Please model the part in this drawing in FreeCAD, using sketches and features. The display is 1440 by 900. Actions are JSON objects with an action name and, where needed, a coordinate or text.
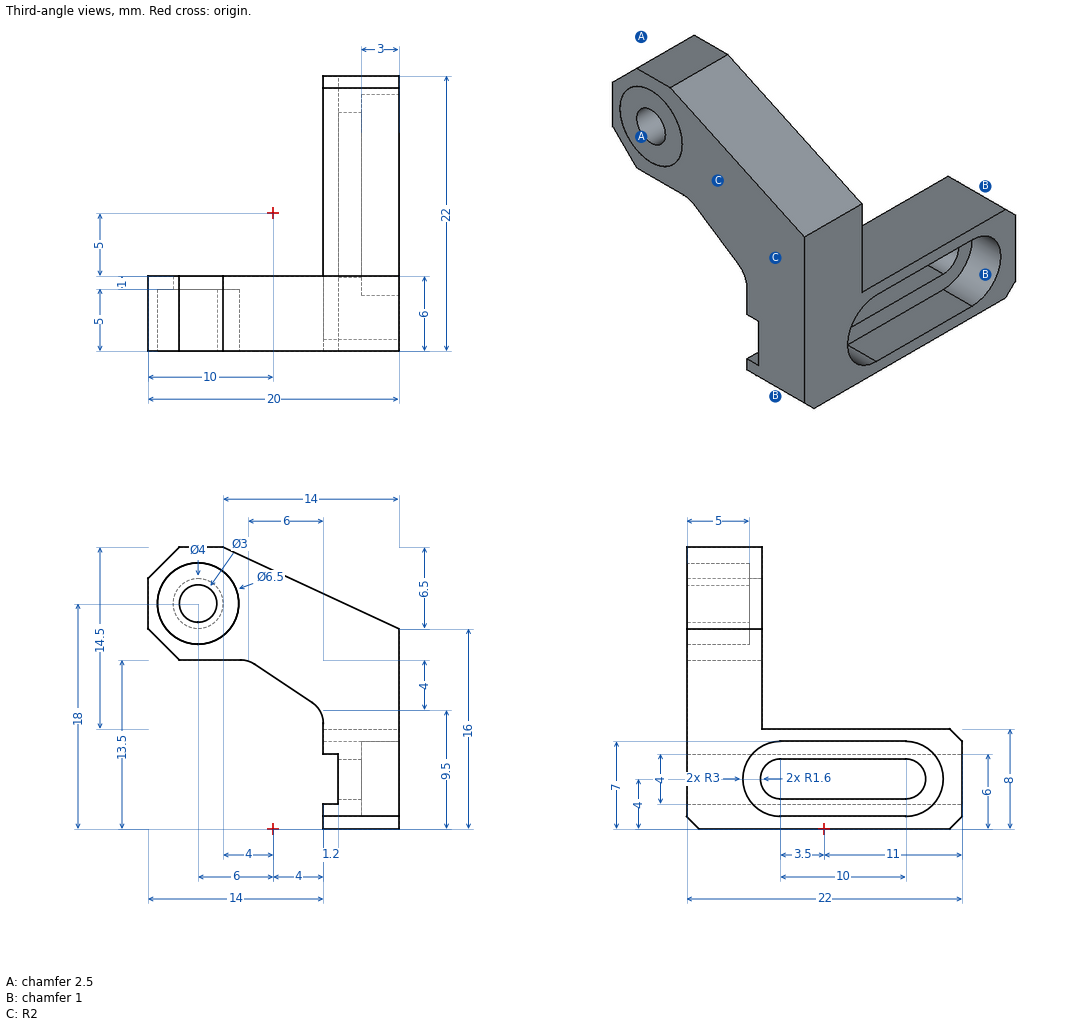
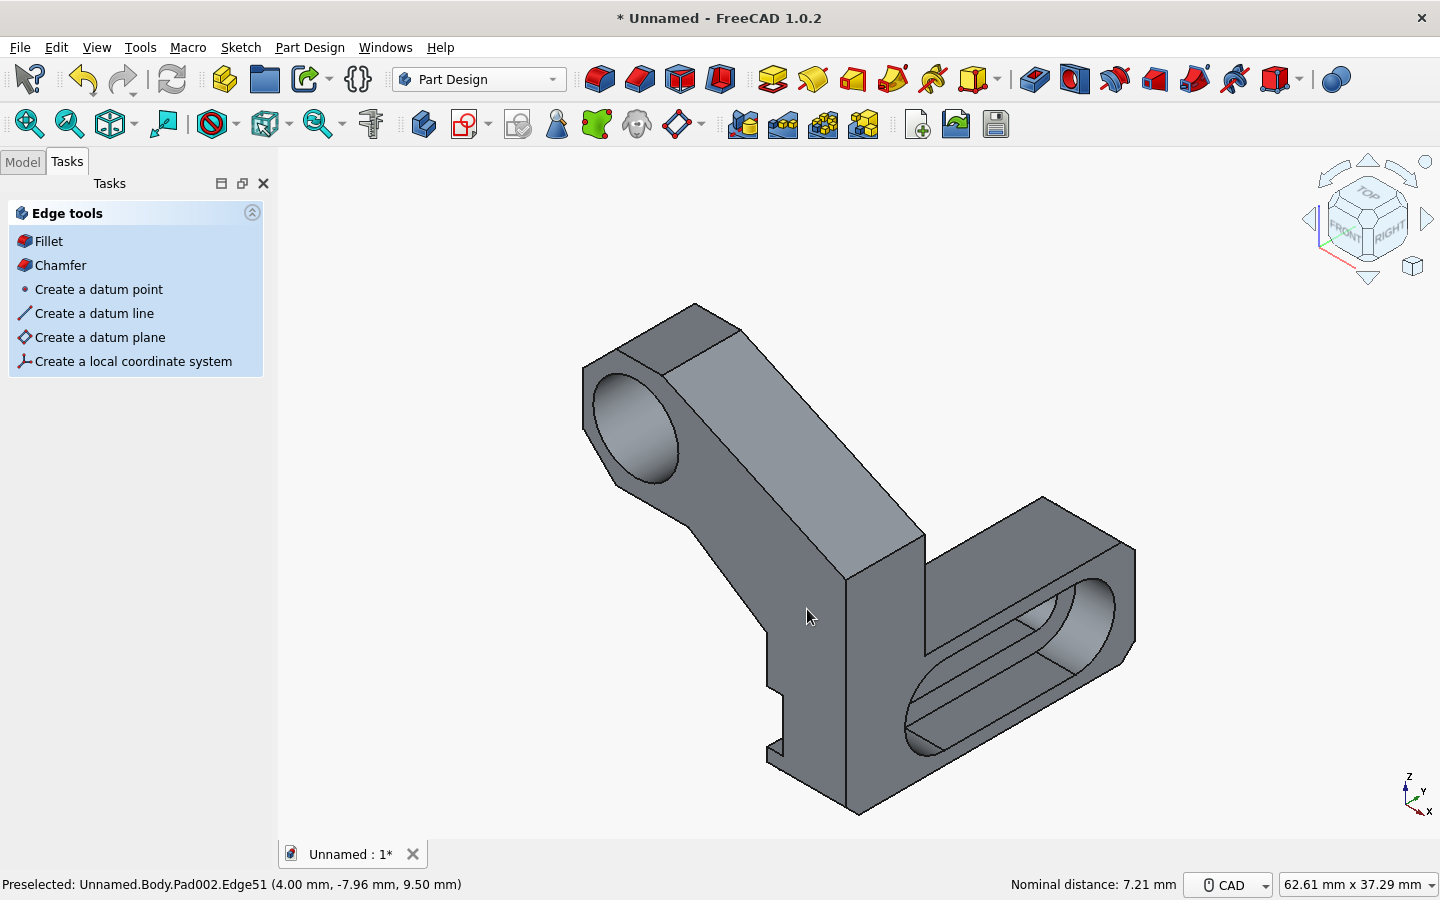
{"action": "left_click", "coordinate": [600, 80]}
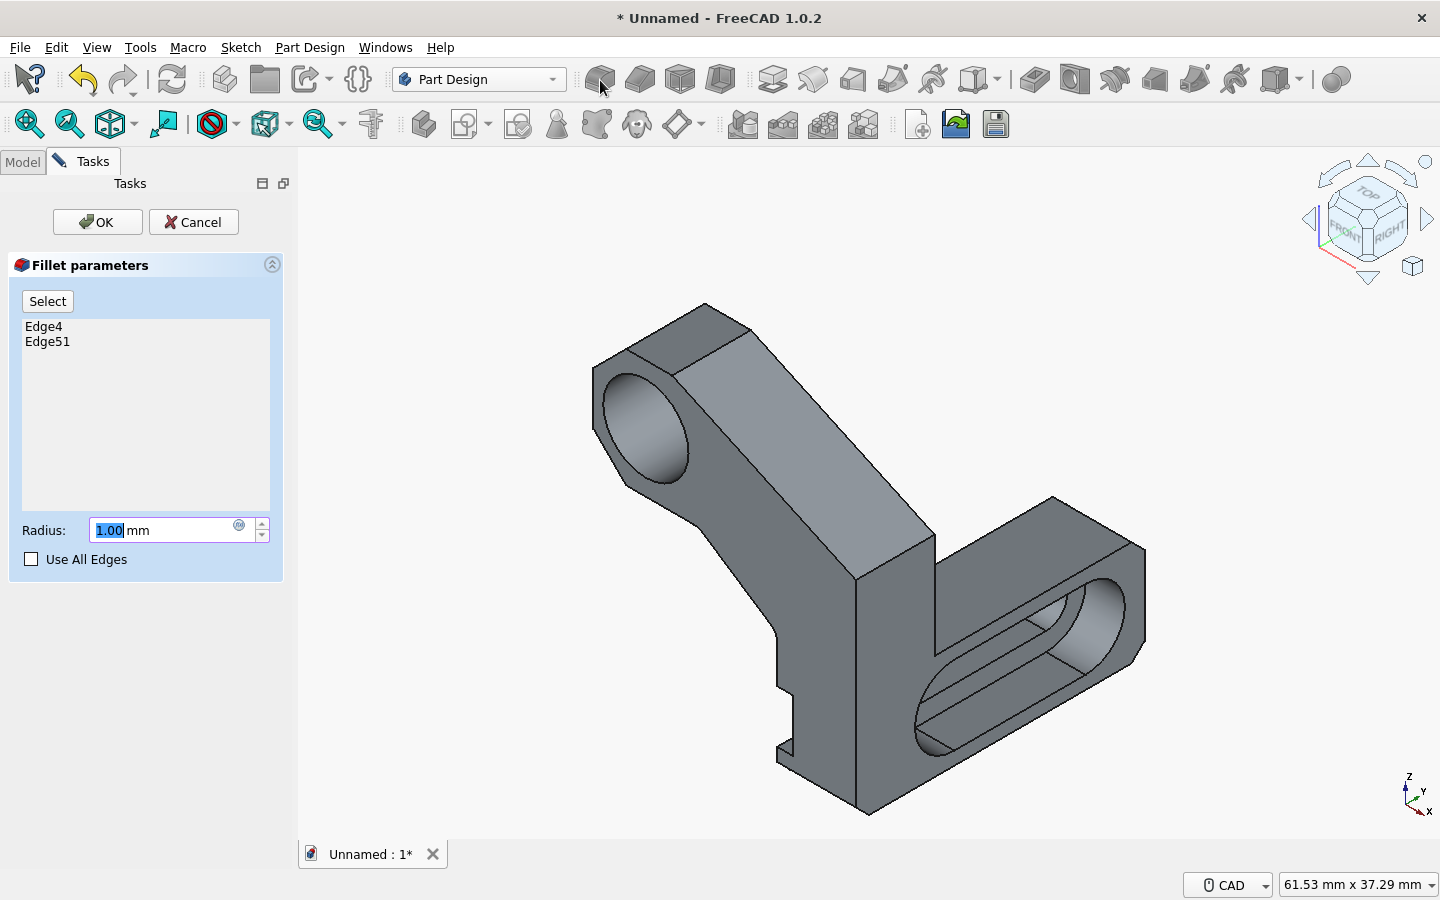
{"action": "type", "text": "2"}
{"action": "key", "text": "Tab"}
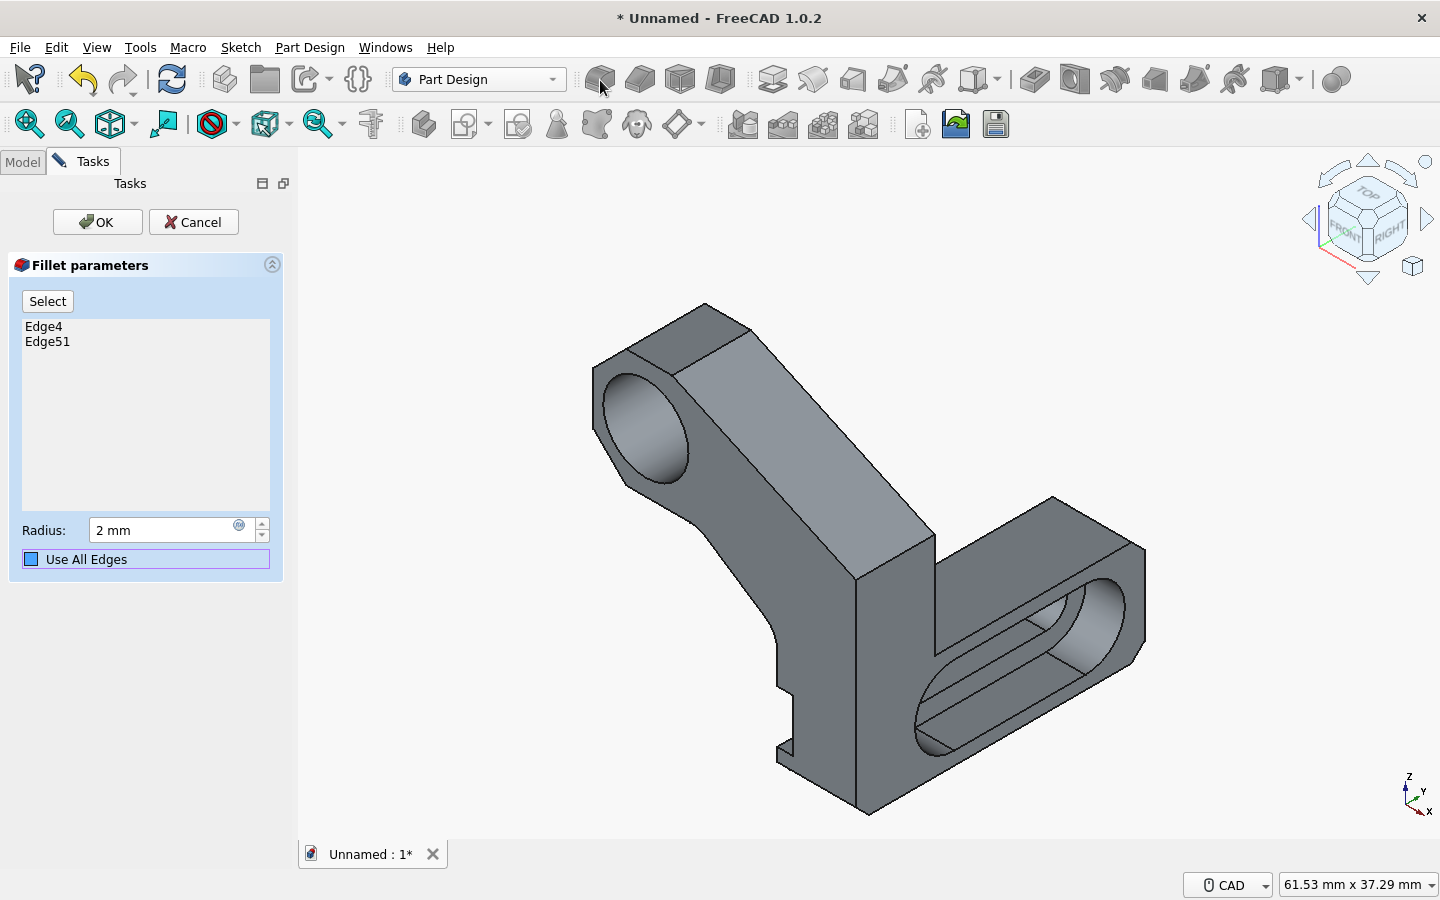
{"action": "left_click", "coordinate": [98, 222]}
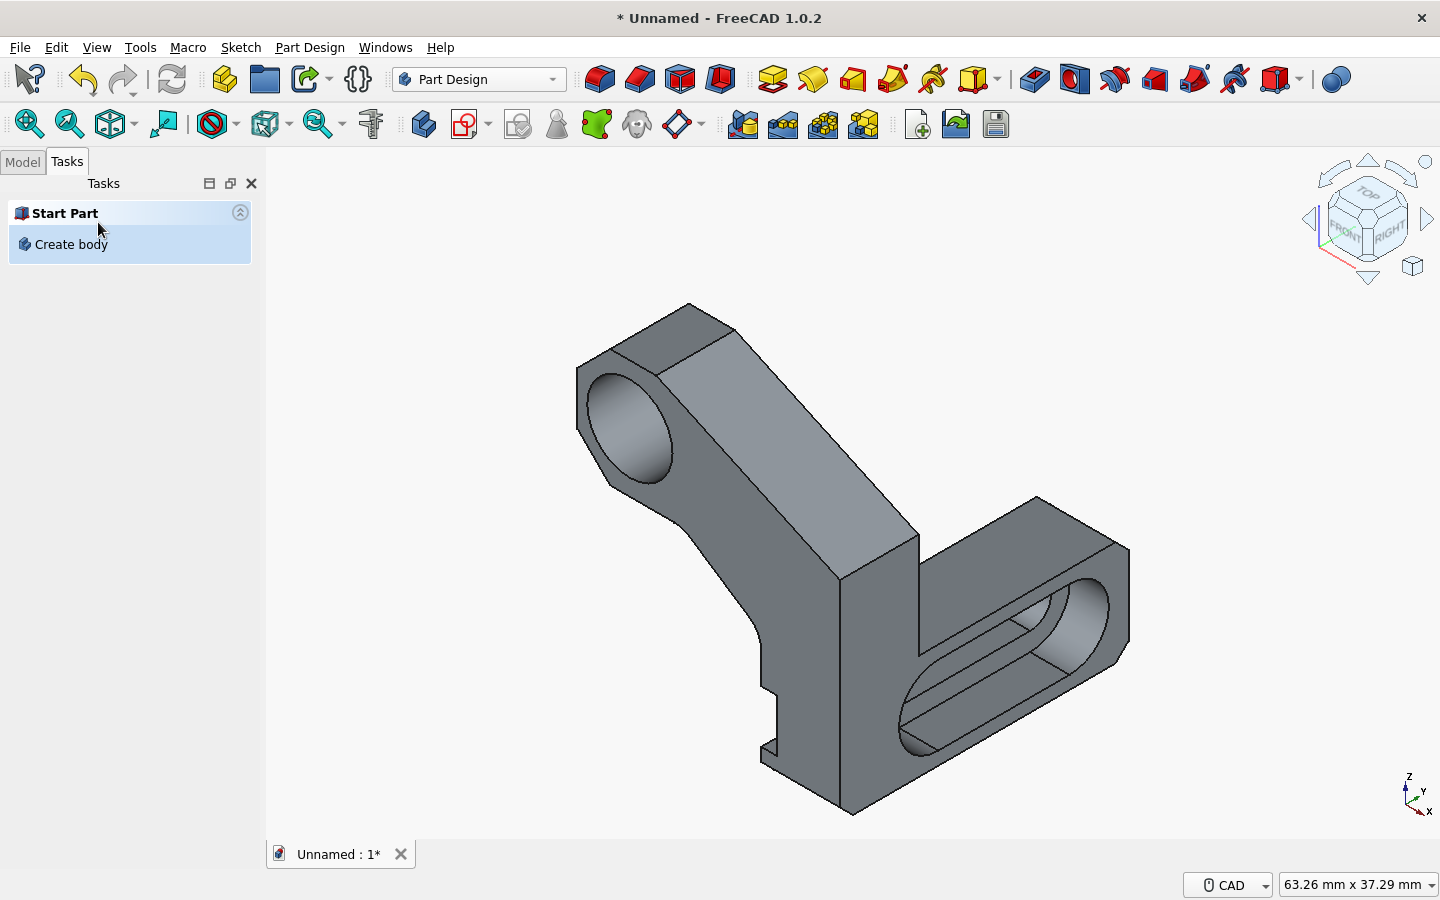
{"action": "left_click", "coordinate": [746, 543]}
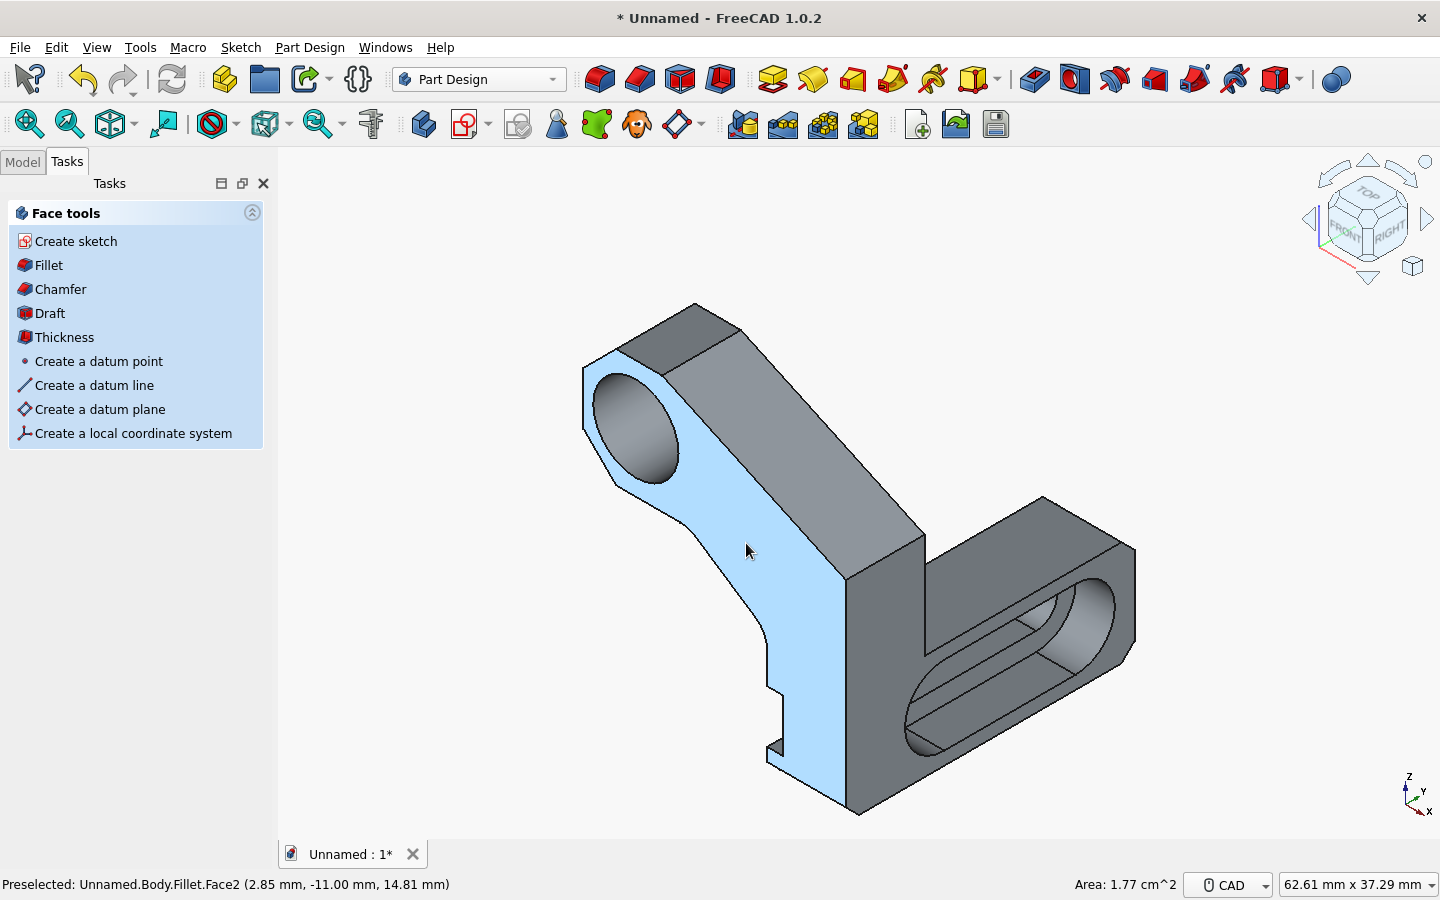
{"action": "left_click", "coordinate": [464, 124]}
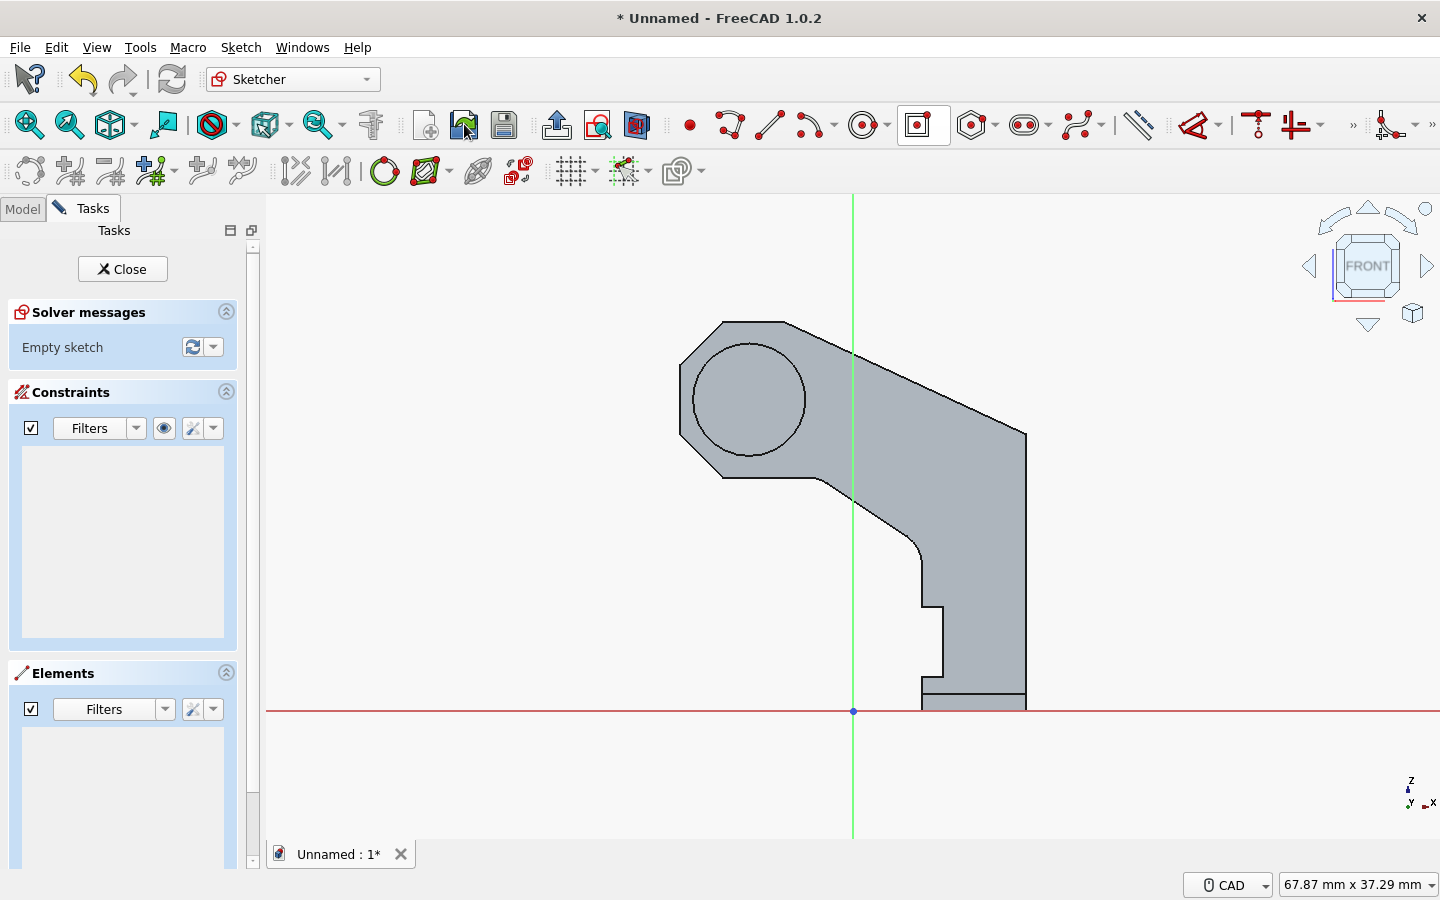
{"action": "scroll", "coordinate": [744, 381], "scroll_direction": "up", "scroll_amount": 10}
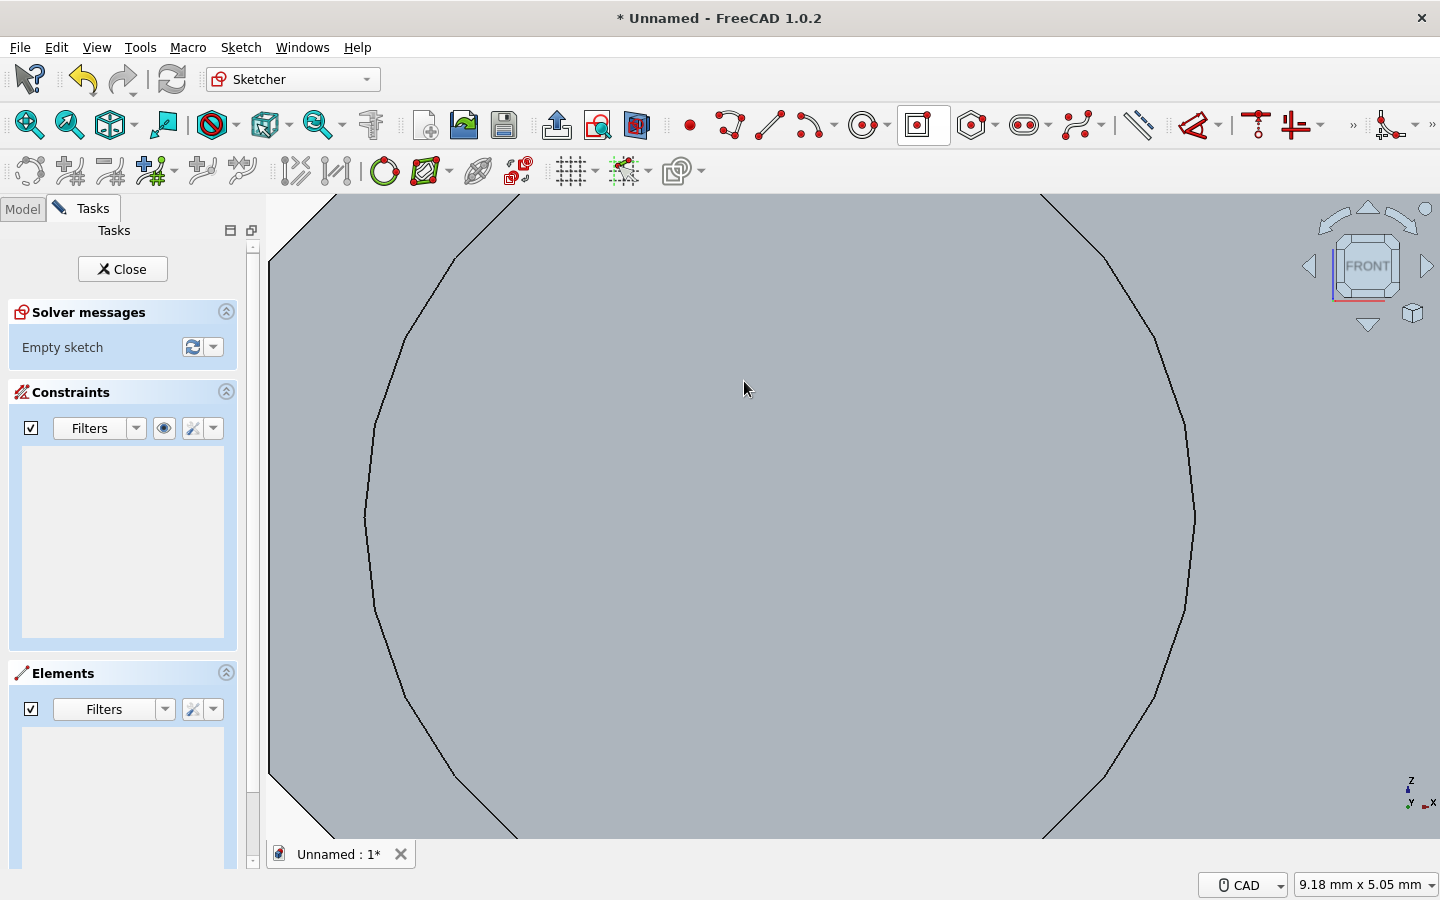
{"action": "left_click", "coordinate": [864, 126]}